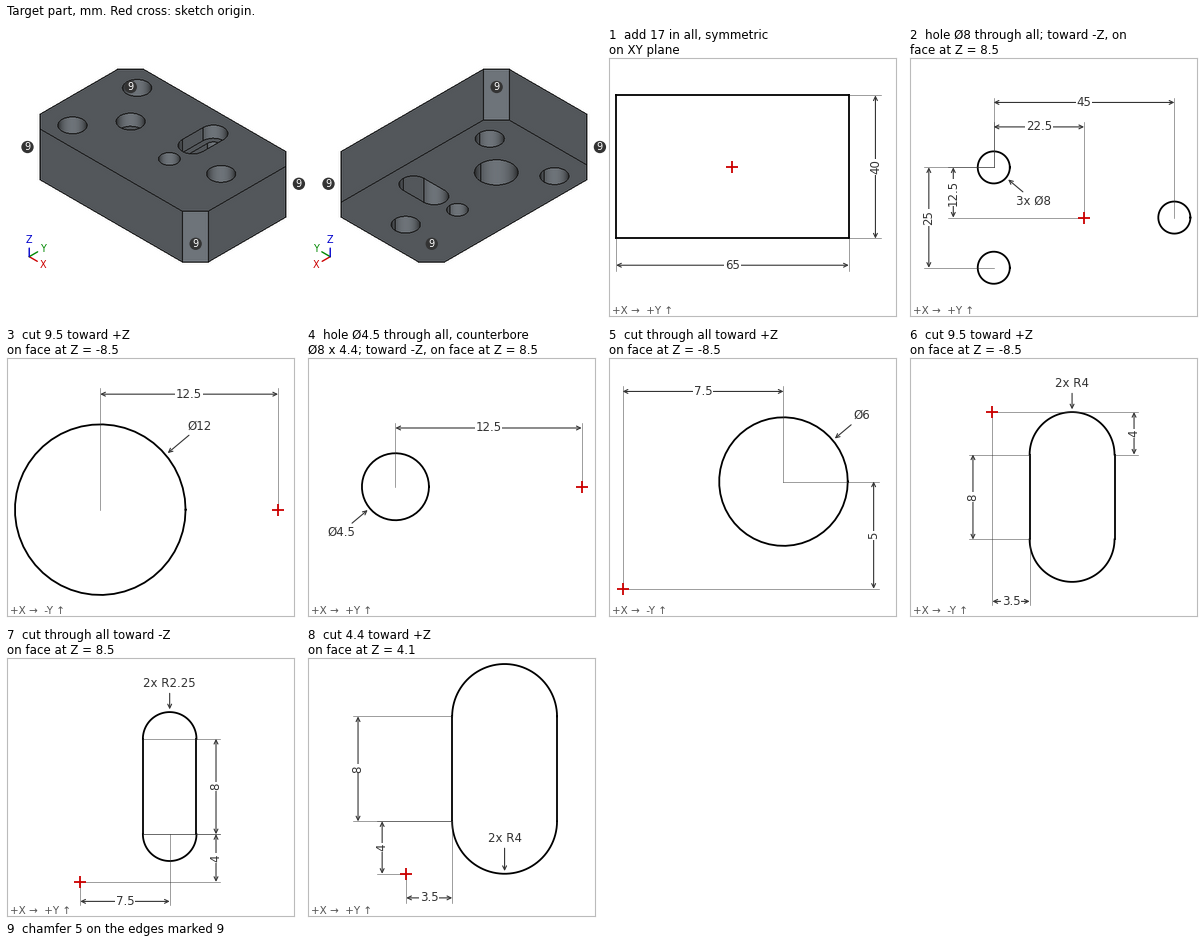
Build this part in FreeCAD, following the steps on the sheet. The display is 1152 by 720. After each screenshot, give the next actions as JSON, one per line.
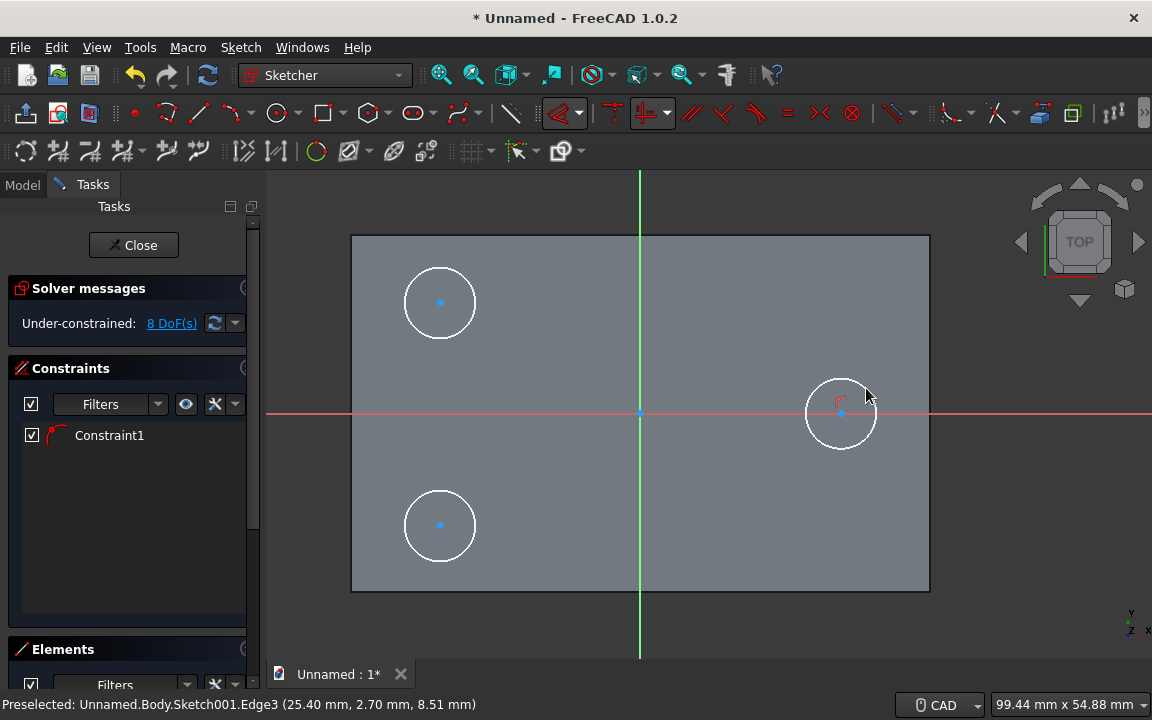
{"action": "left_click", "coordinate": [465, 278]}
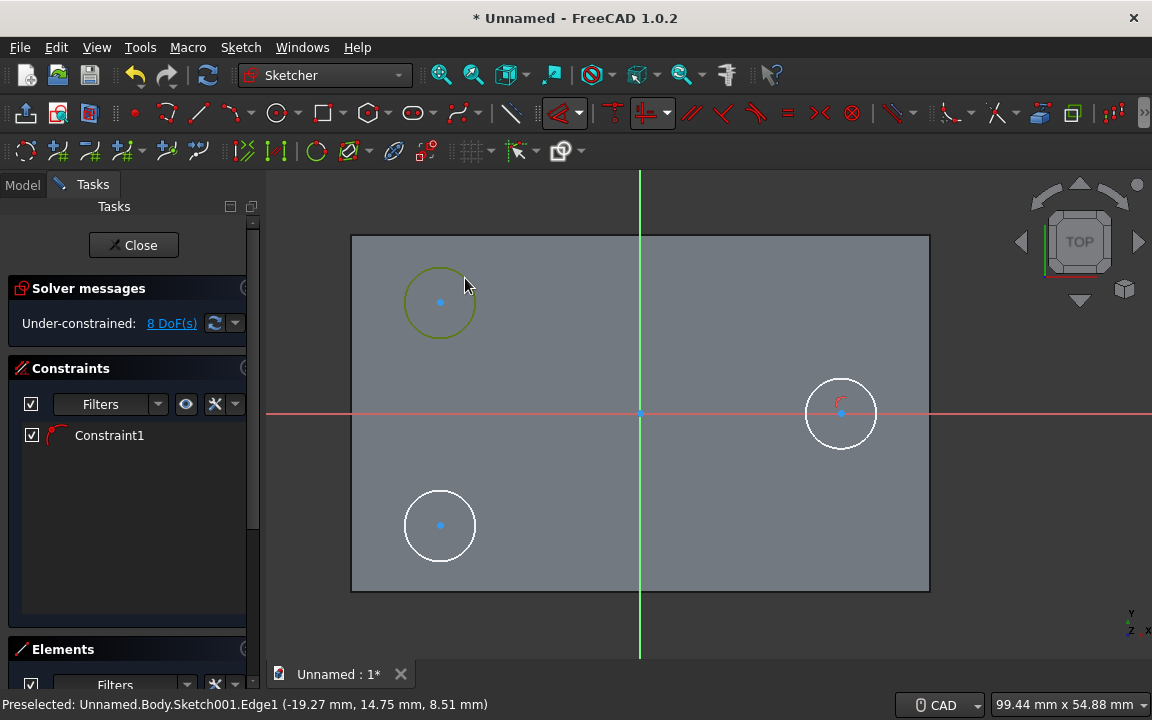
{"action": "left_click", "coordinate": [465, 501]}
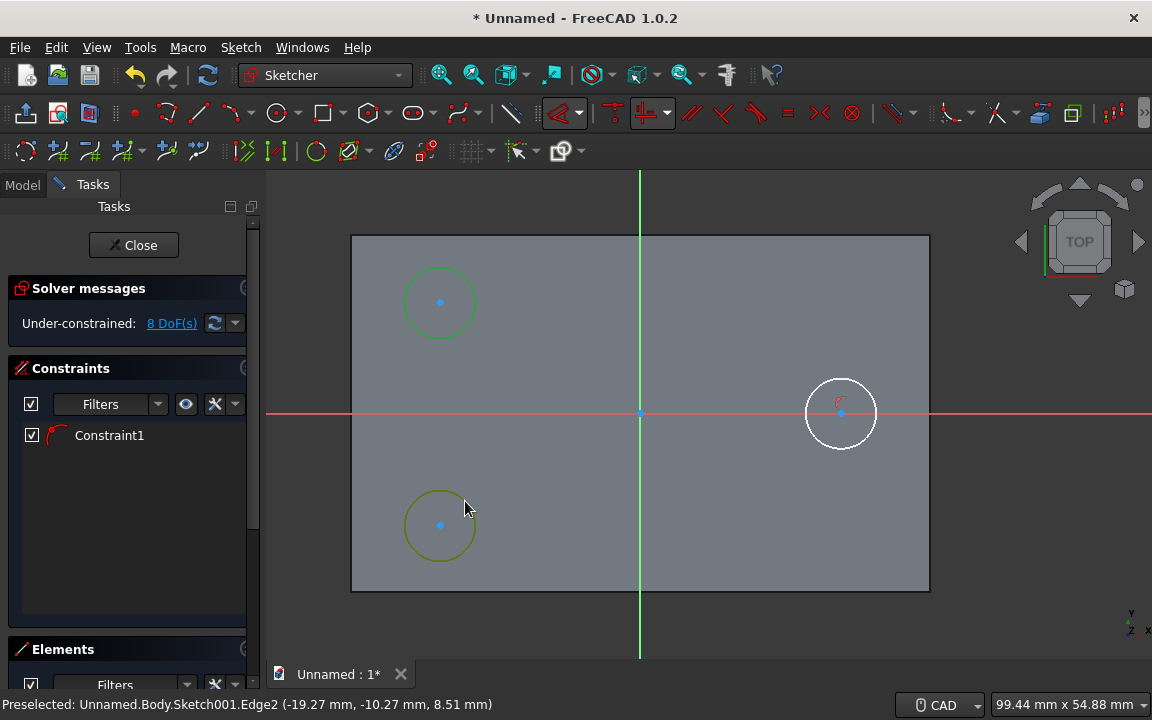
{"action": "left_click", "coordinate": [866, 389]}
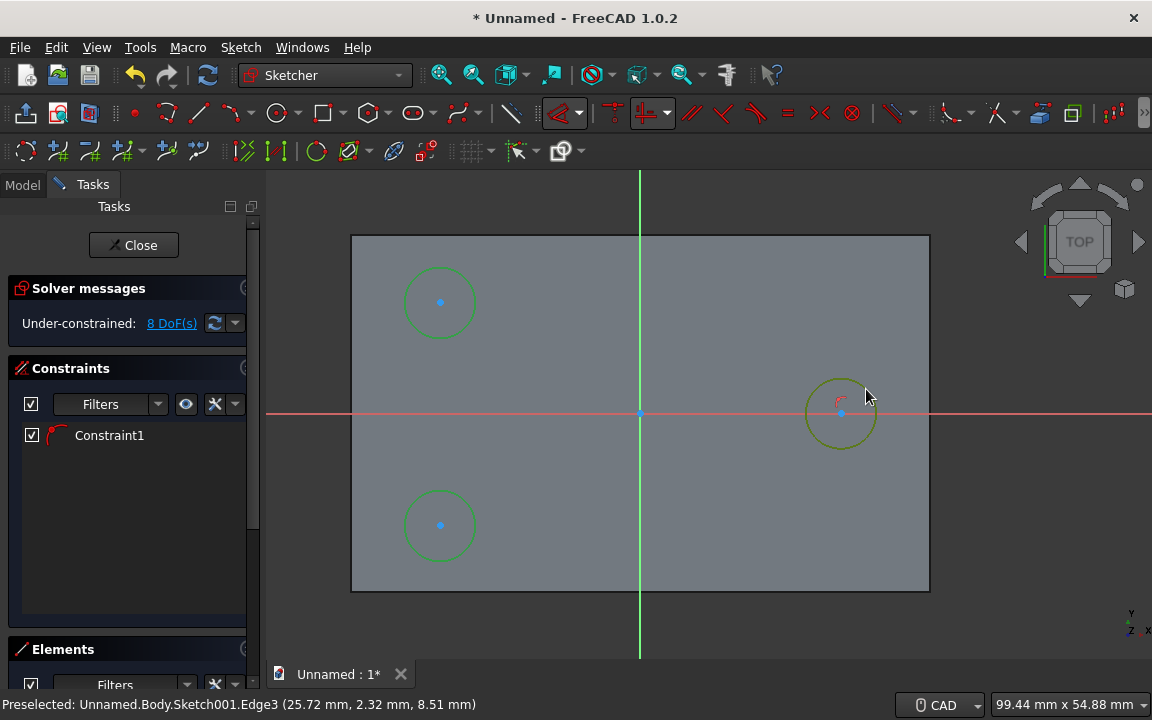
{"action": "left_click", "coordinate": [788, 114]}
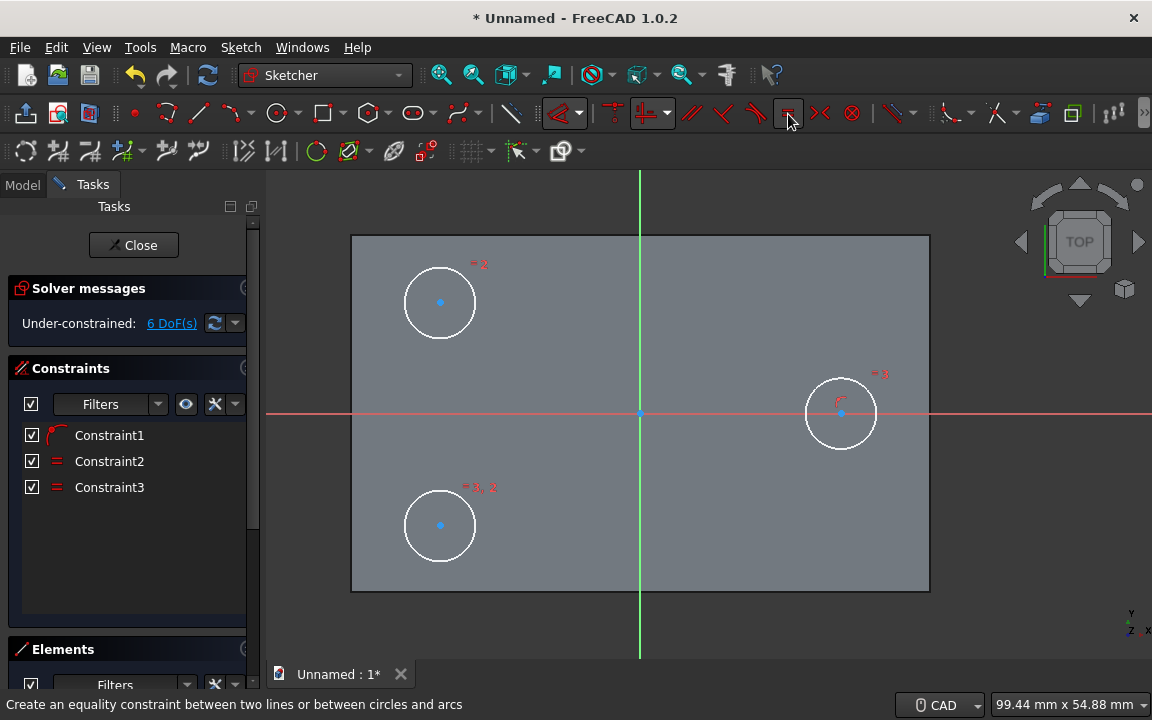
{"action": "left_click", "coordinate": [440, 303]}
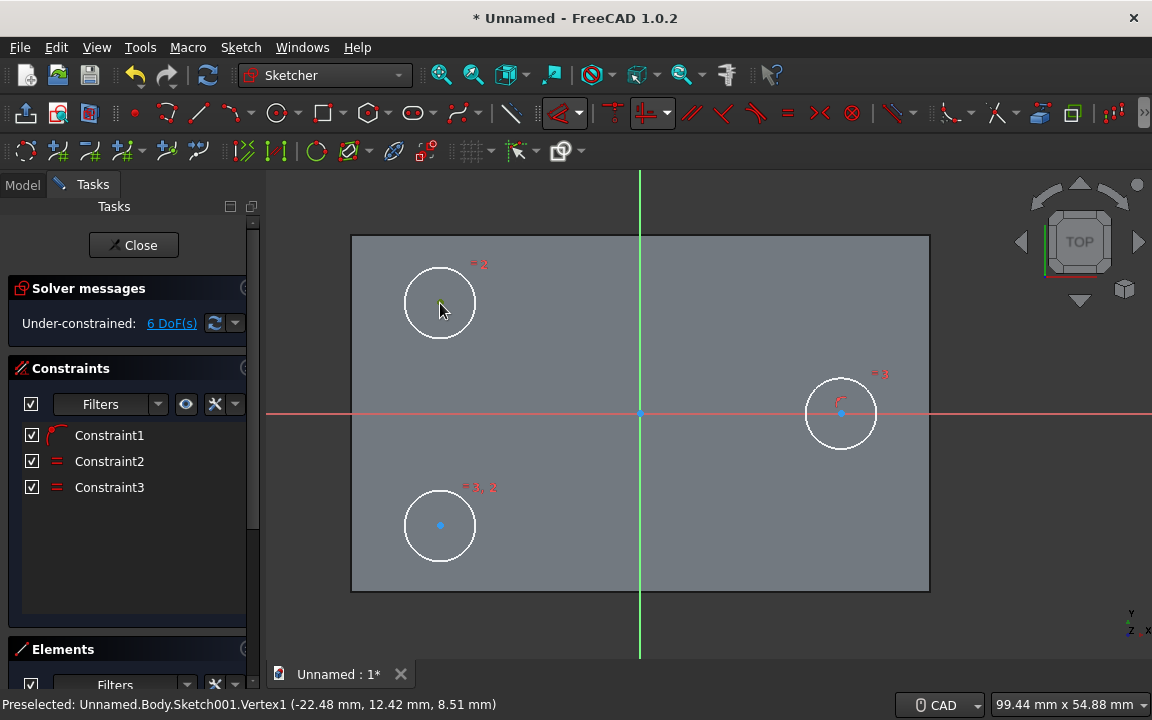
{"action": "left_click", "coordinate": [440, 526]}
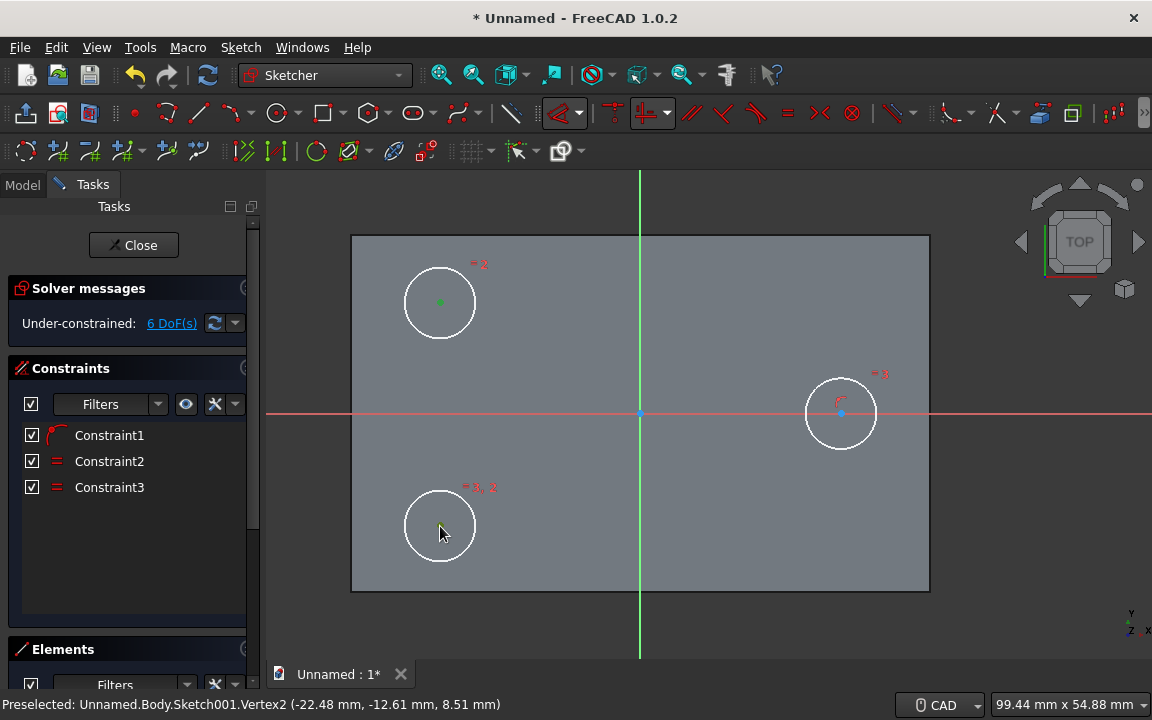
{"action": "left_click", "coordinate": [670, 114]}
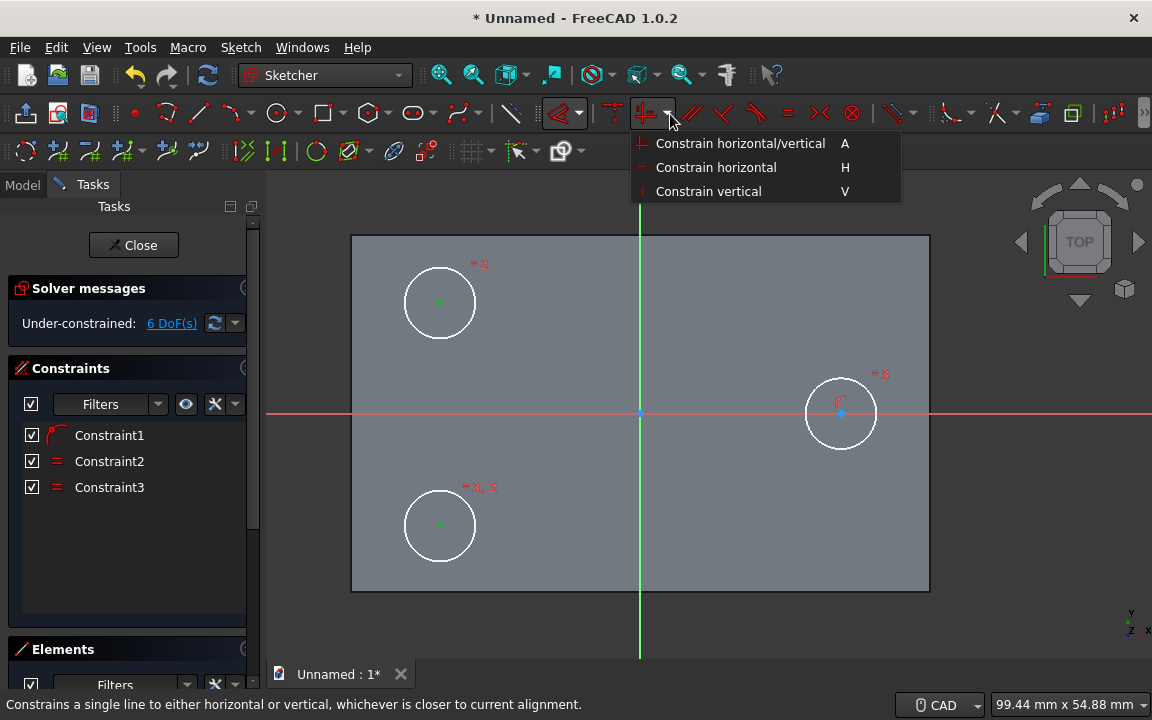
{"action": "left_click", "coordinate": [766, 191]}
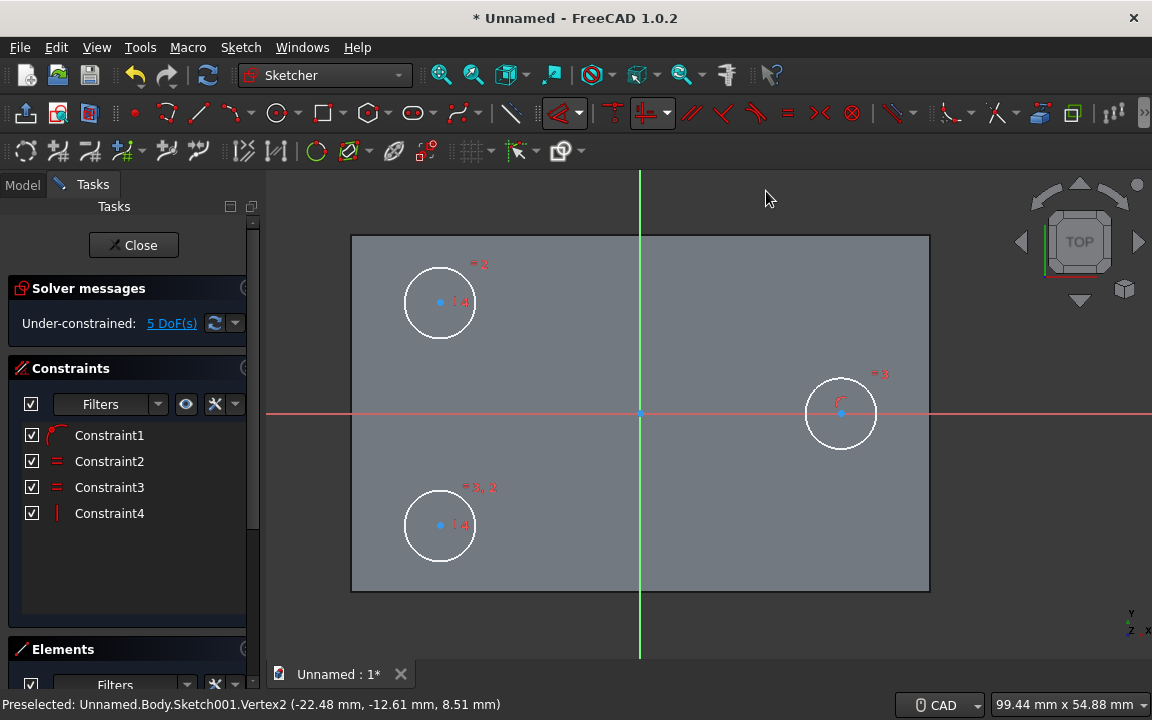
{"action": "key", "text": "d"}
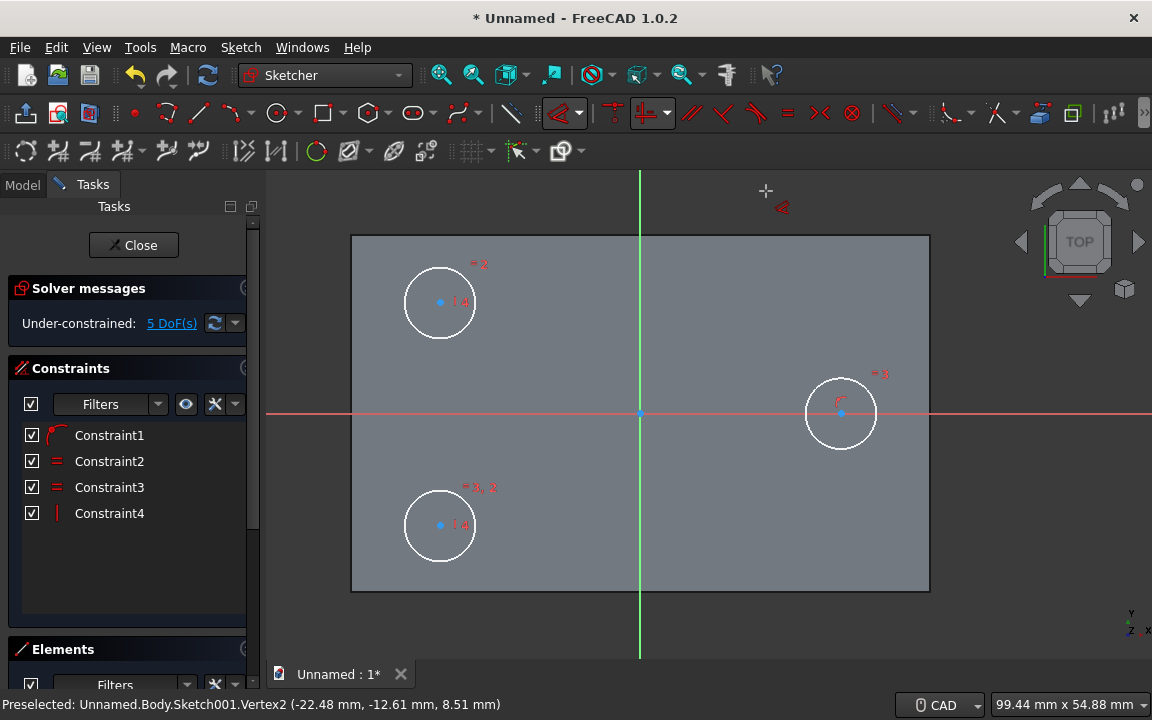
{"action": "left_click", "coordinate": [465, 278]}
{"action": "left_click", "coordinate": [488, 255]}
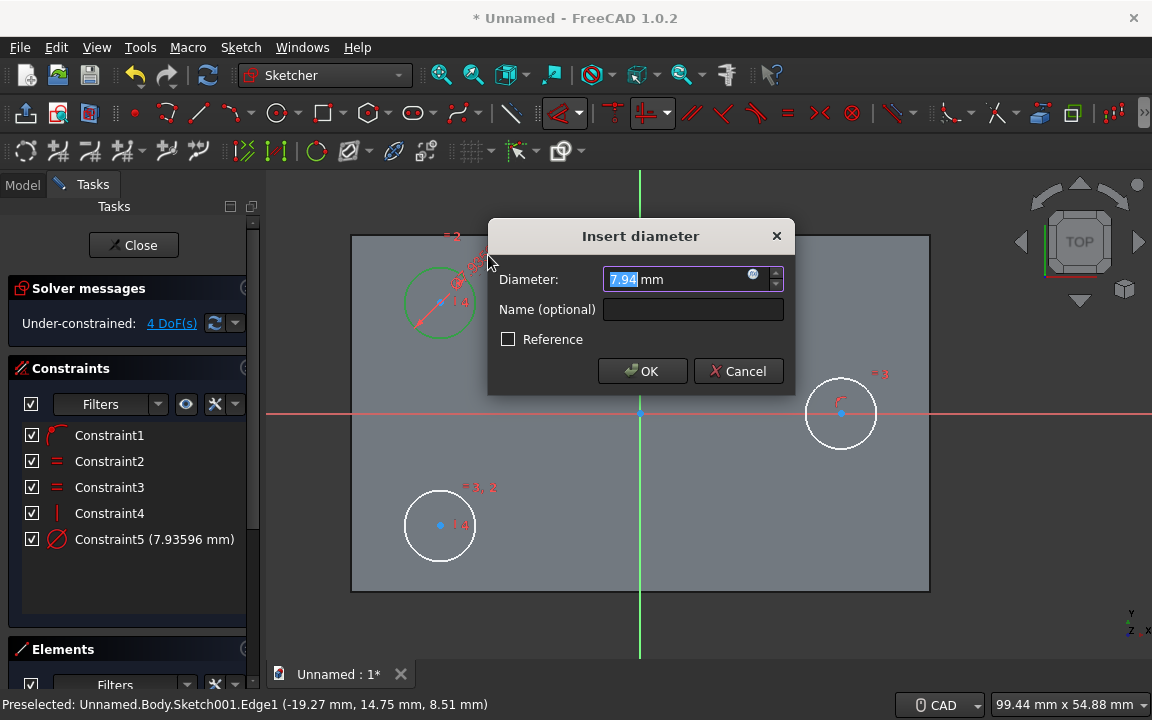
{"action": "type", "text": "8"}
{"action": "key", "text": "Return"}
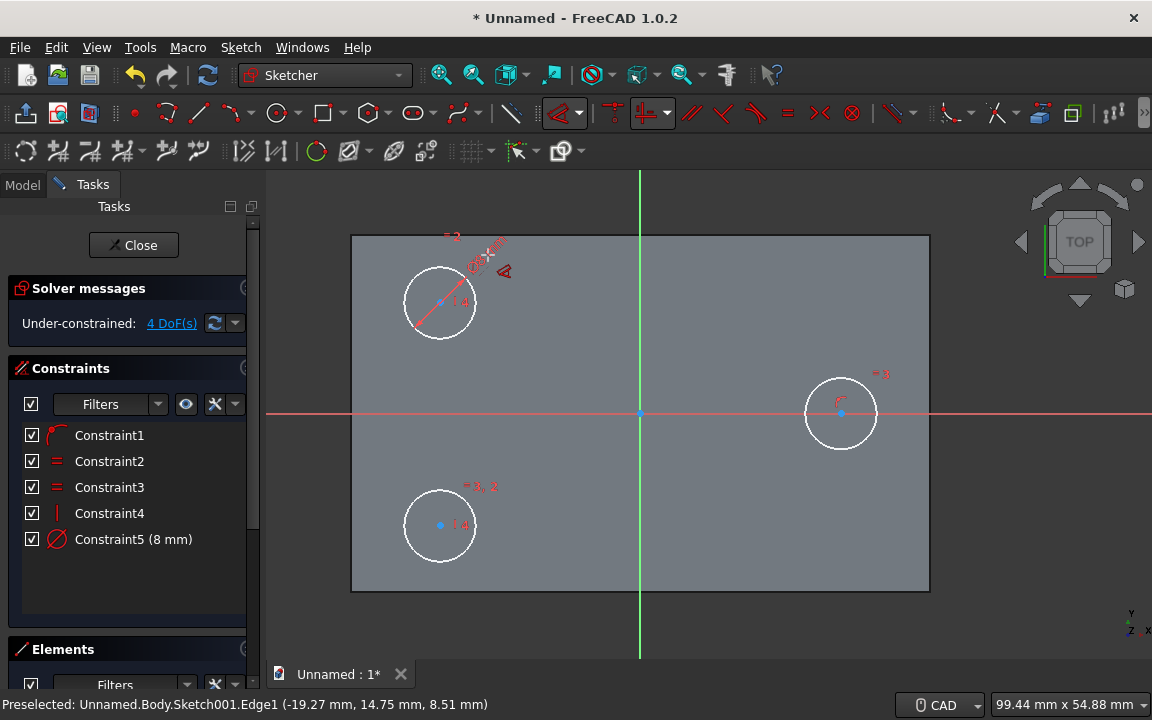
{"action": "left_click", "coordinate": [440, 303]}